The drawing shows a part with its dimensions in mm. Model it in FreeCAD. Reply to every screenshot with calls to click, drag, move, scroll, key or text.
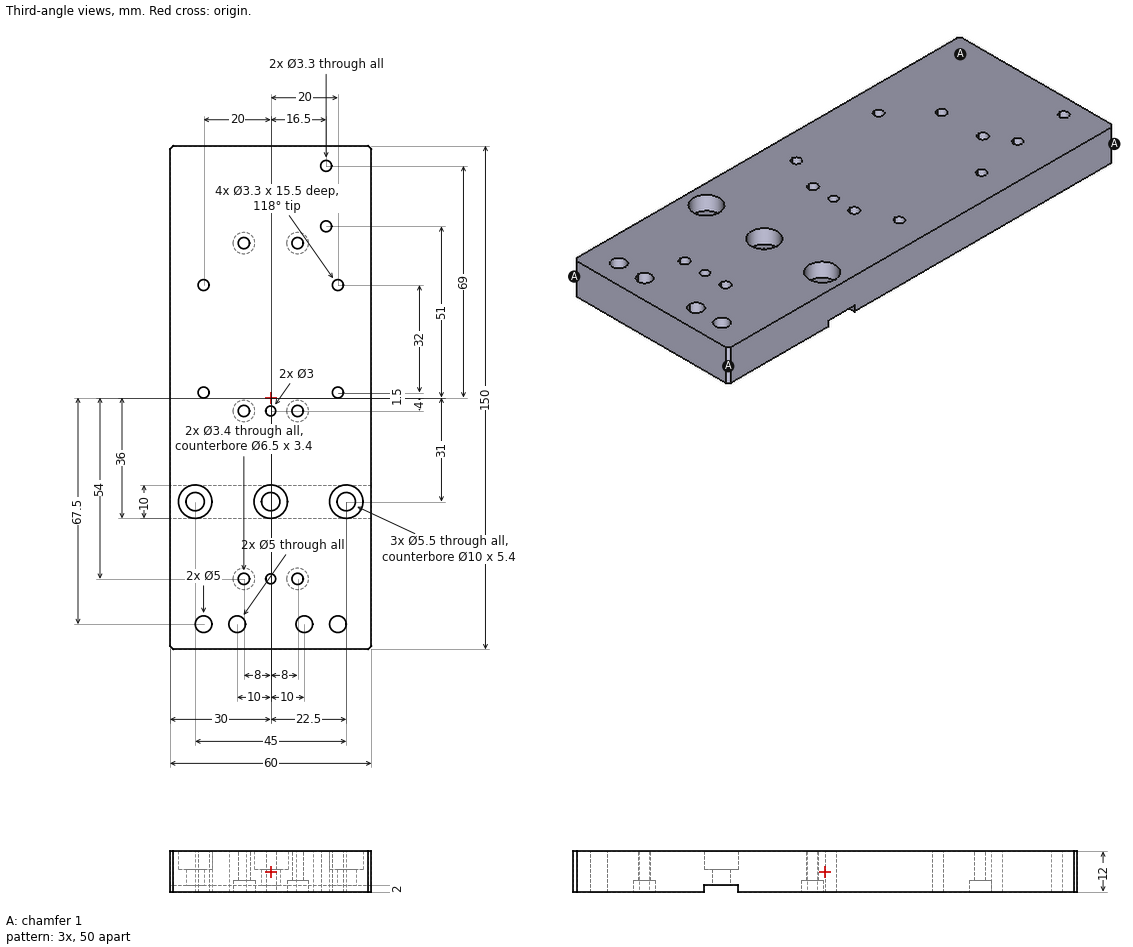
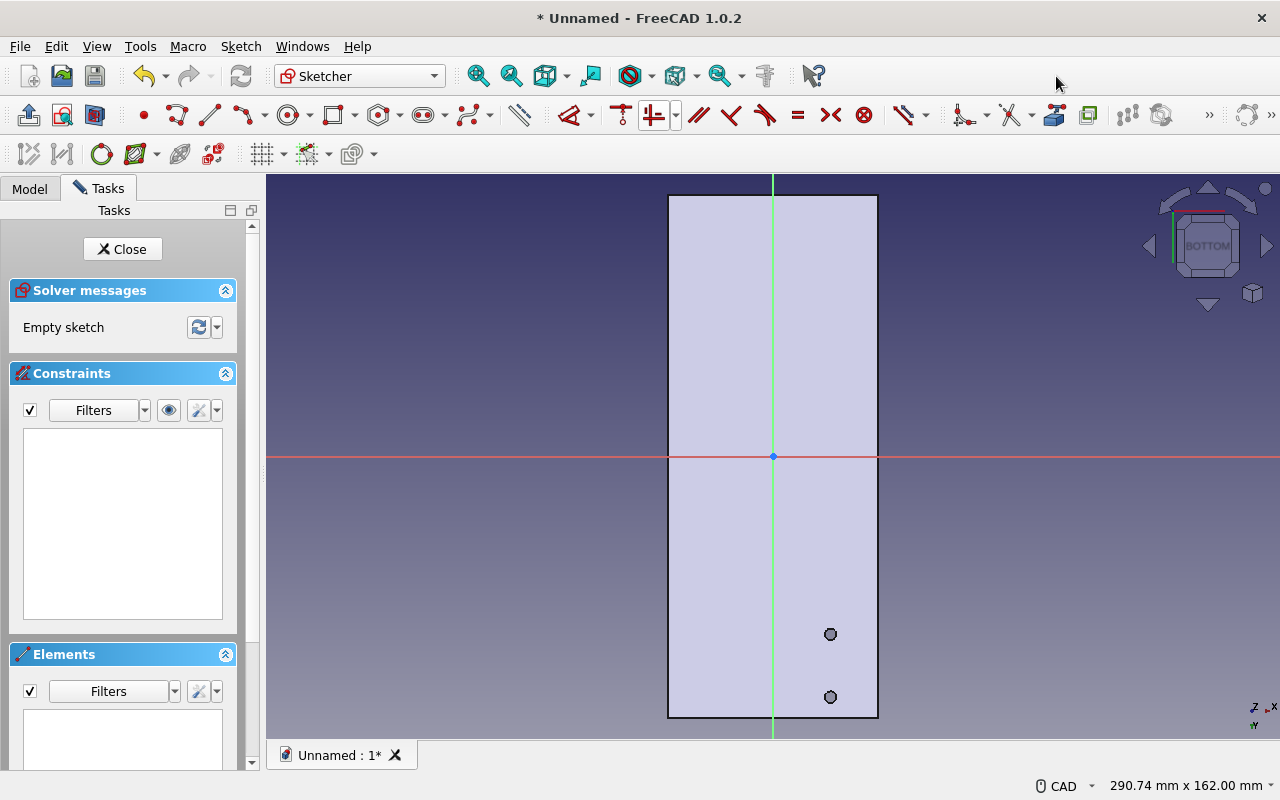
scroll(813, 553, up, 5)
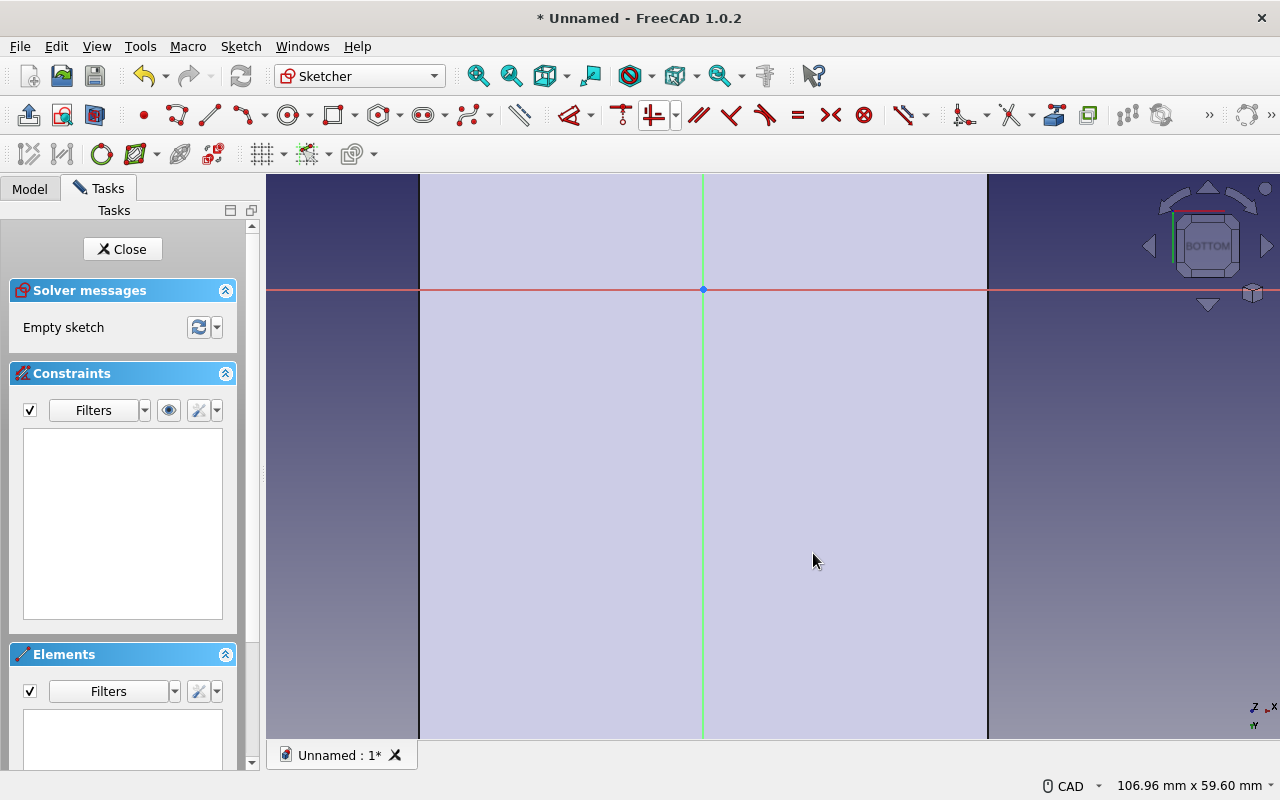
click(288, 116)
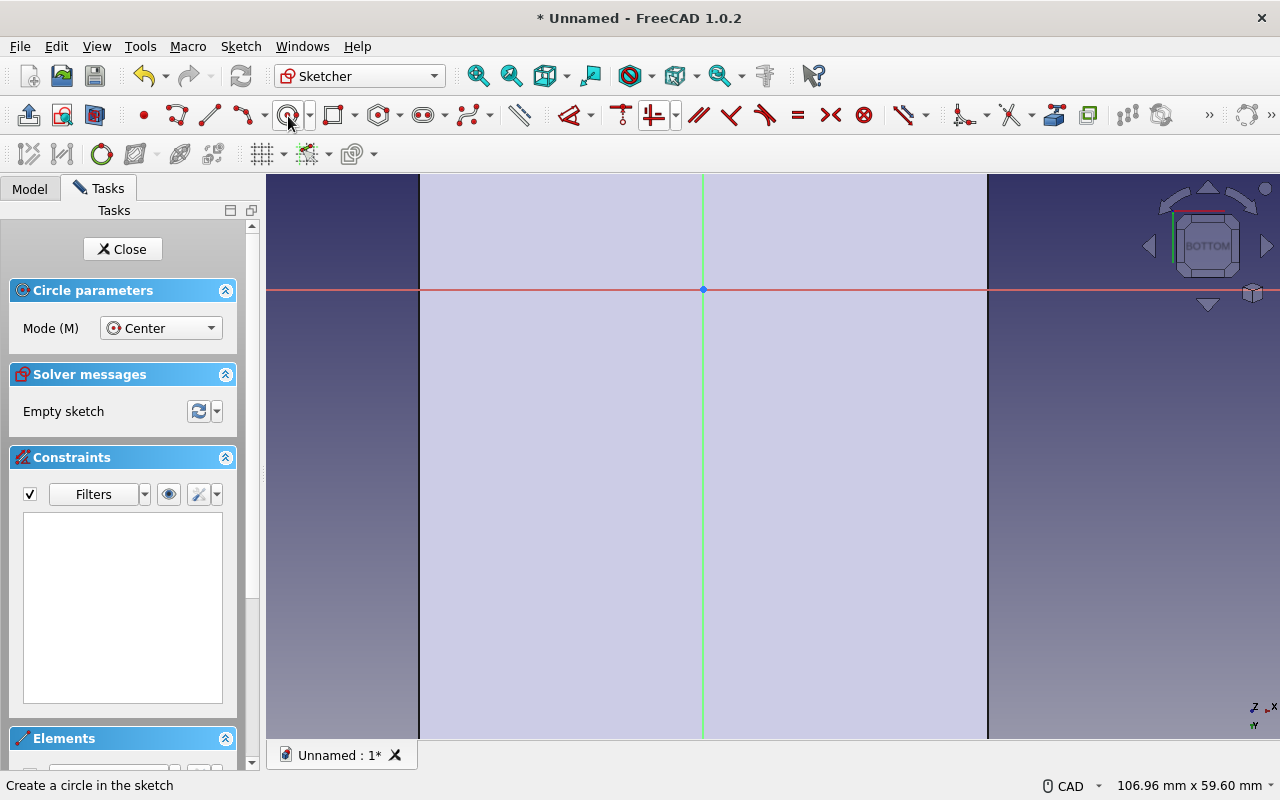
scroll(893, 607, up, 2)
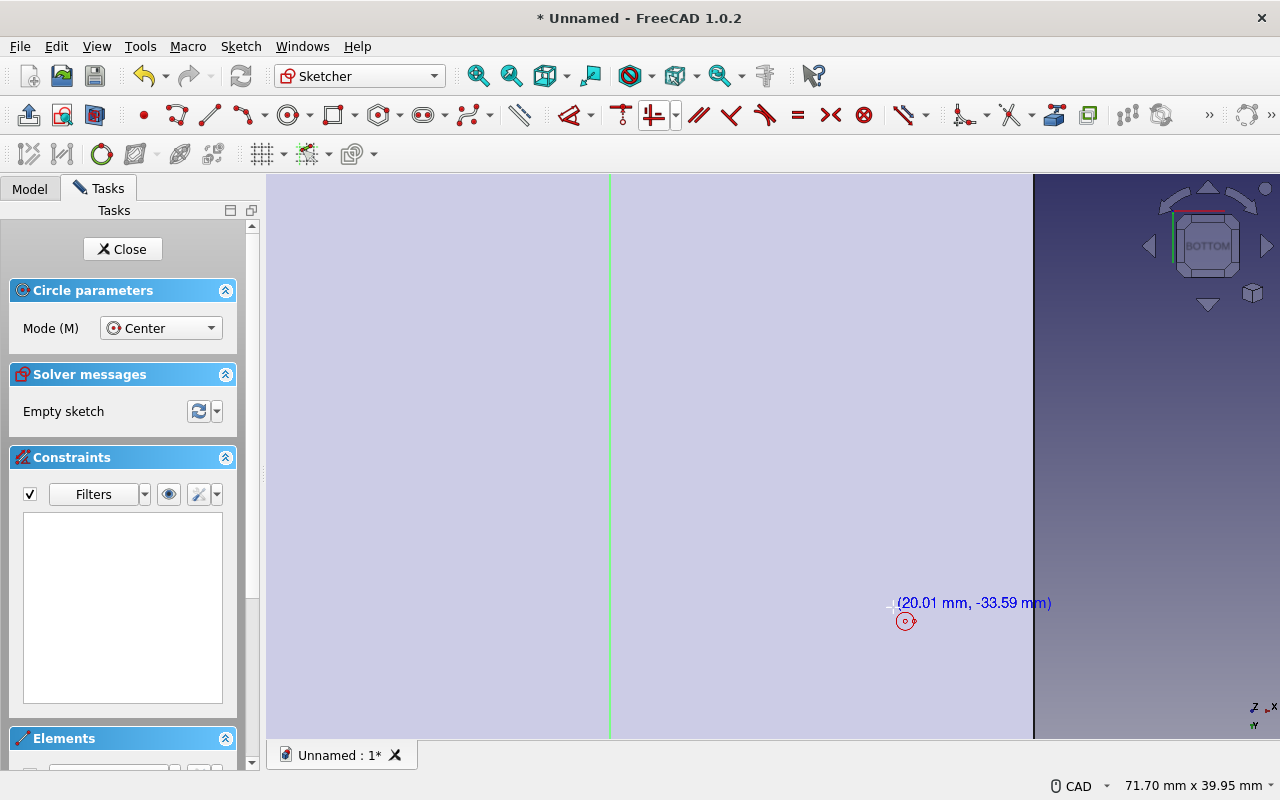
click(893, 607)
click(909, 590)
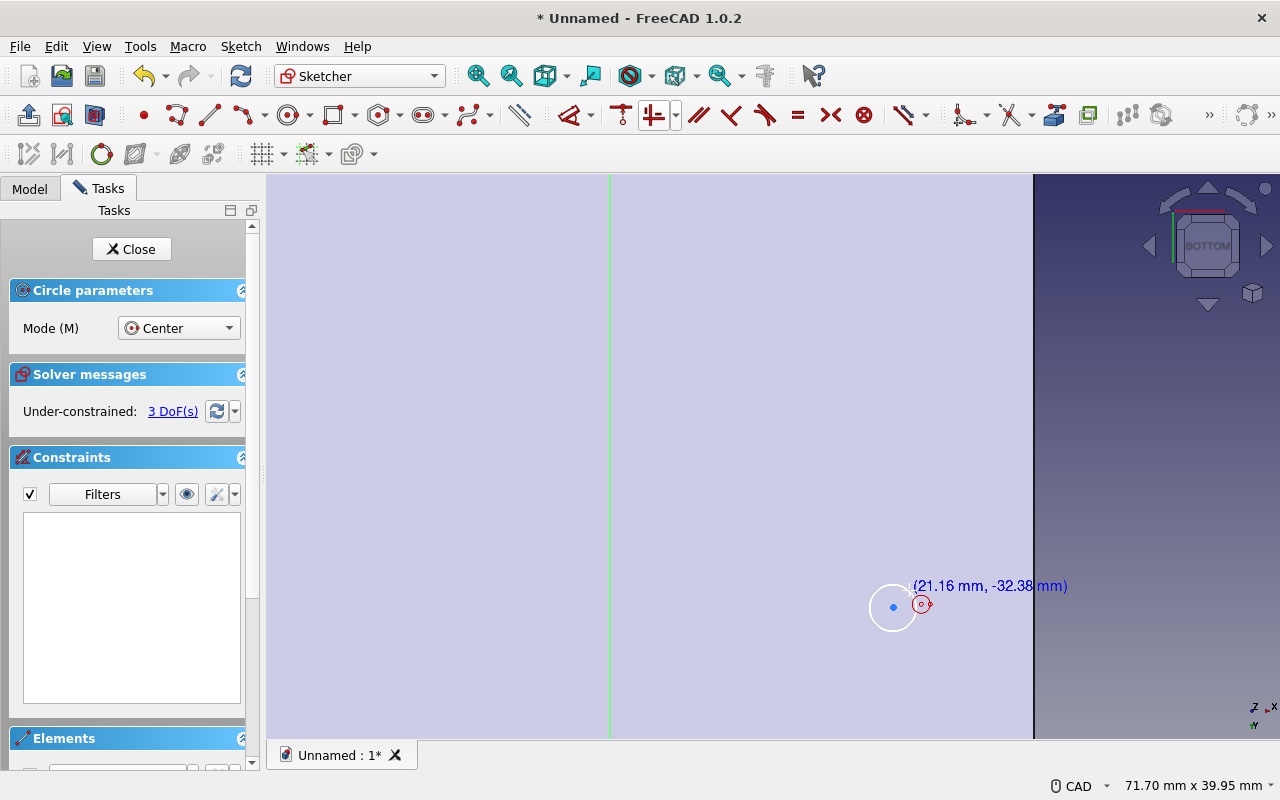
scroll(897, 611, down, 2)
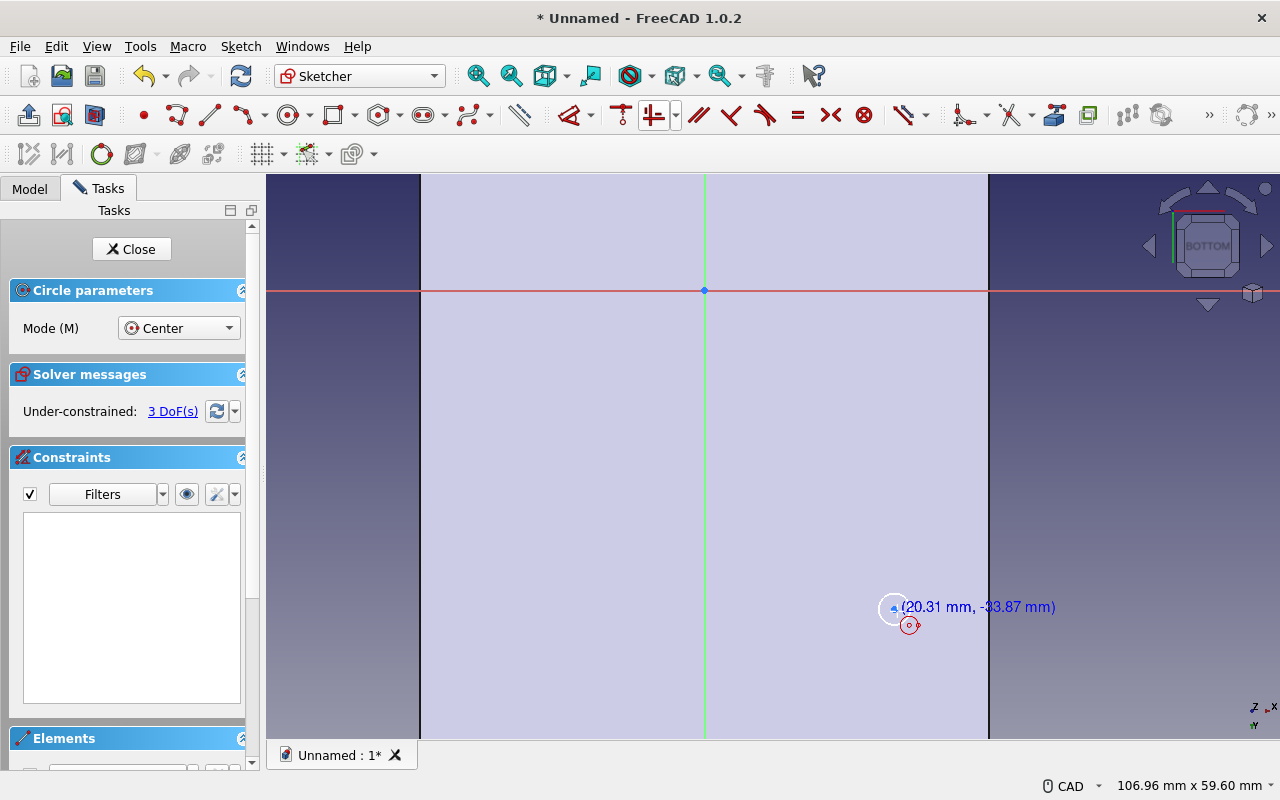
scroll(894, 305, up, 2)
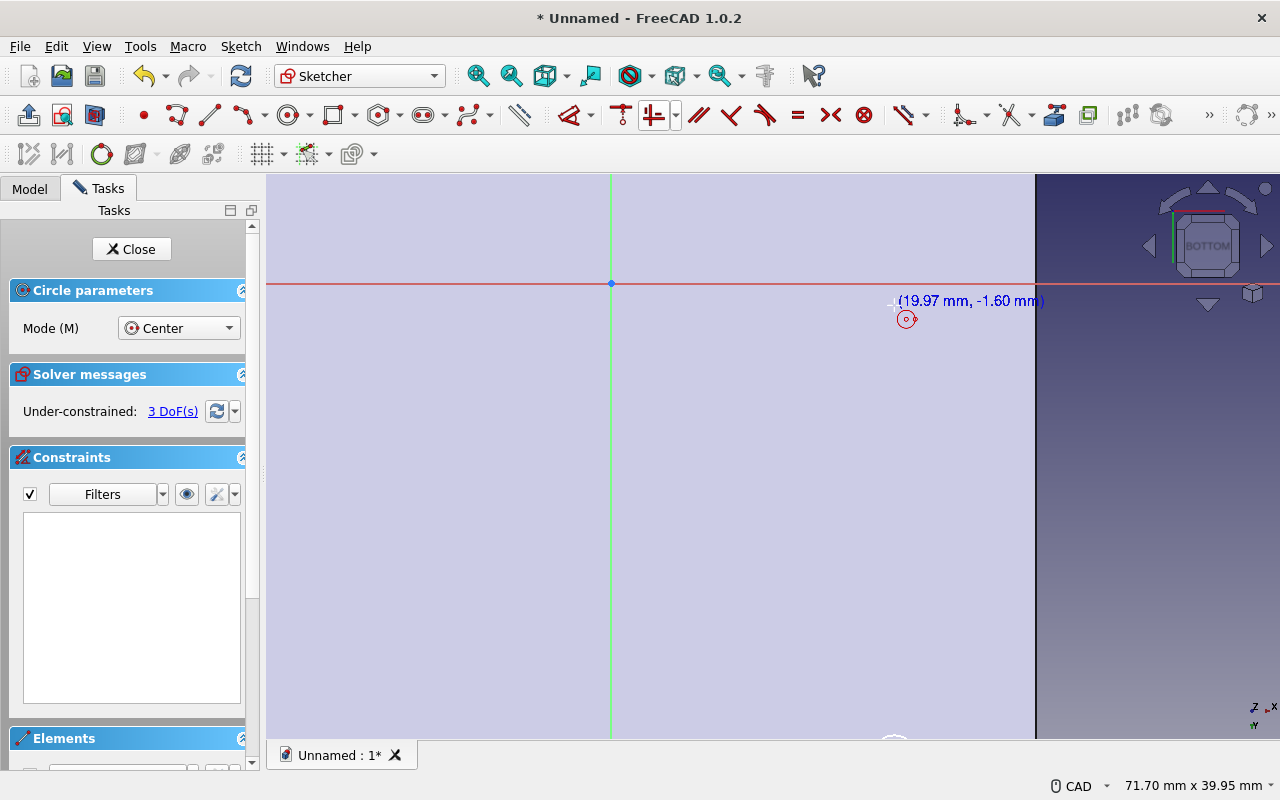
click(894, 305)
click(911, 321)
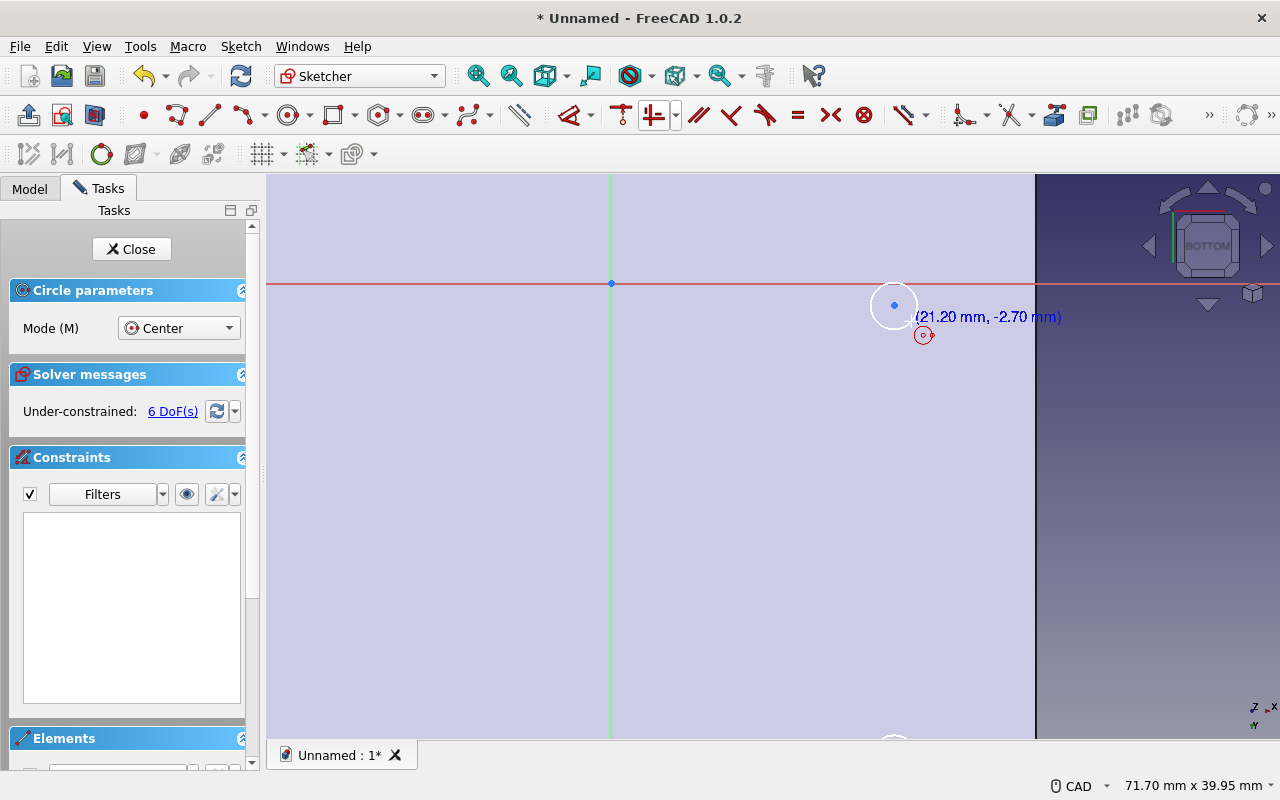
scroll(894, 304, down, 2)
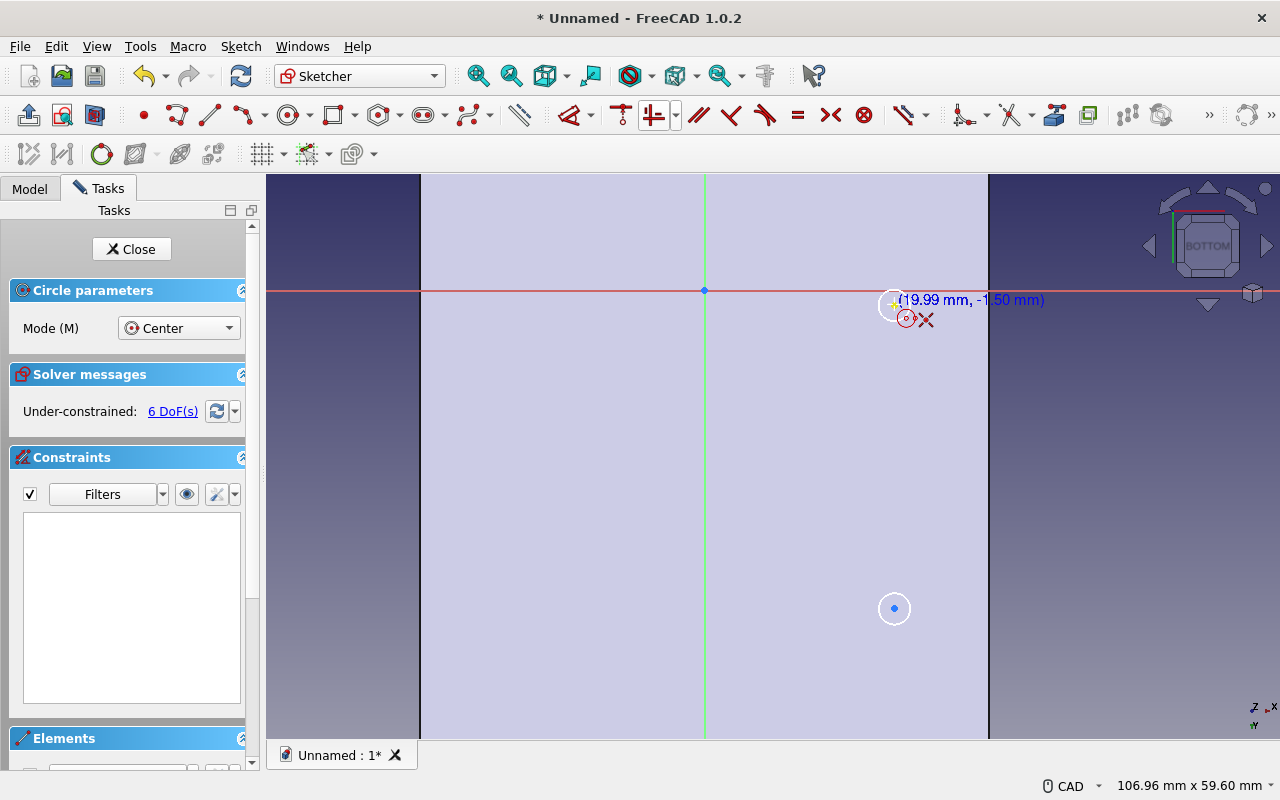
scroll(515, 608, up, 2)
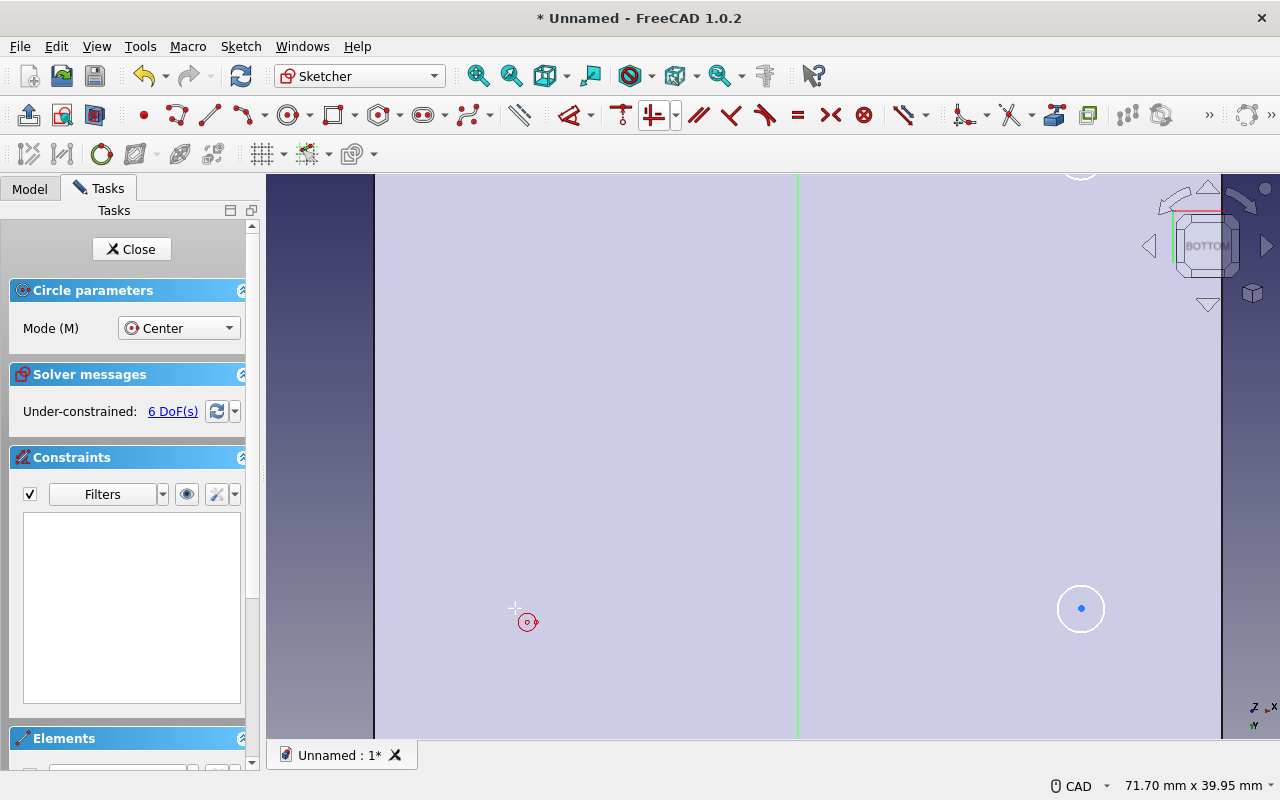
click(515, 608)
click(531, 591)